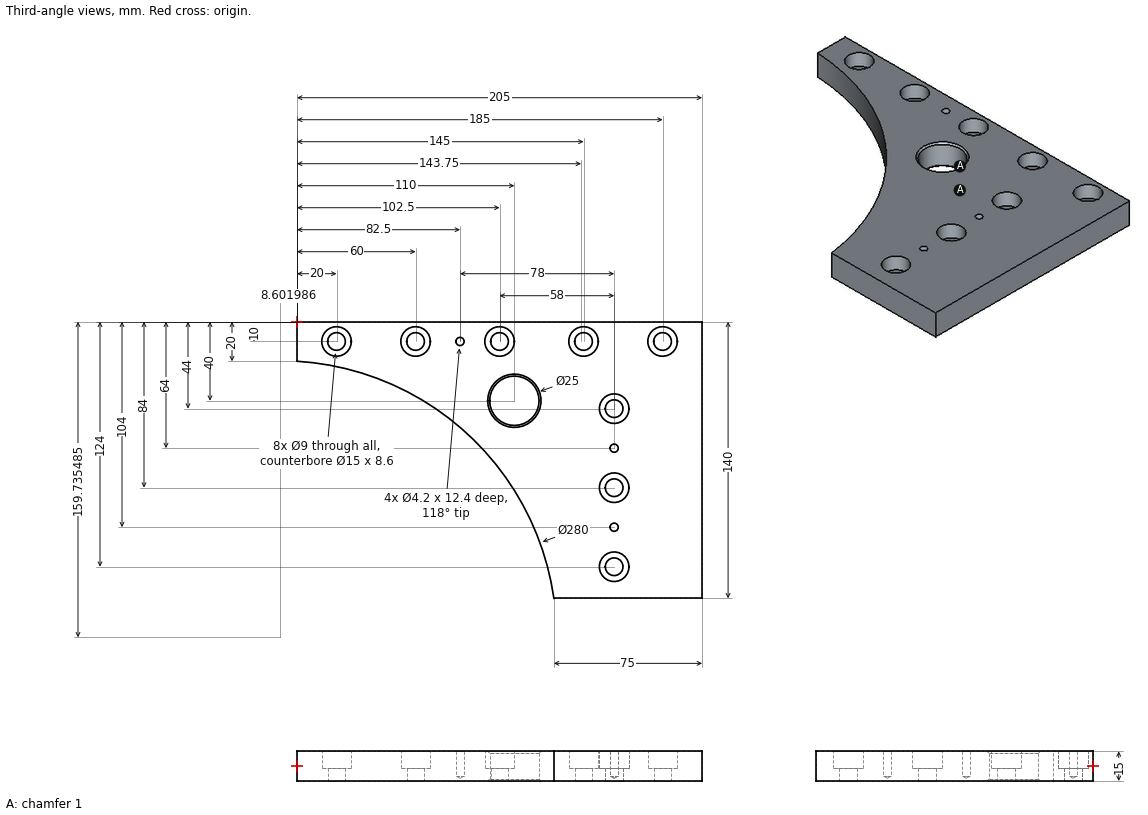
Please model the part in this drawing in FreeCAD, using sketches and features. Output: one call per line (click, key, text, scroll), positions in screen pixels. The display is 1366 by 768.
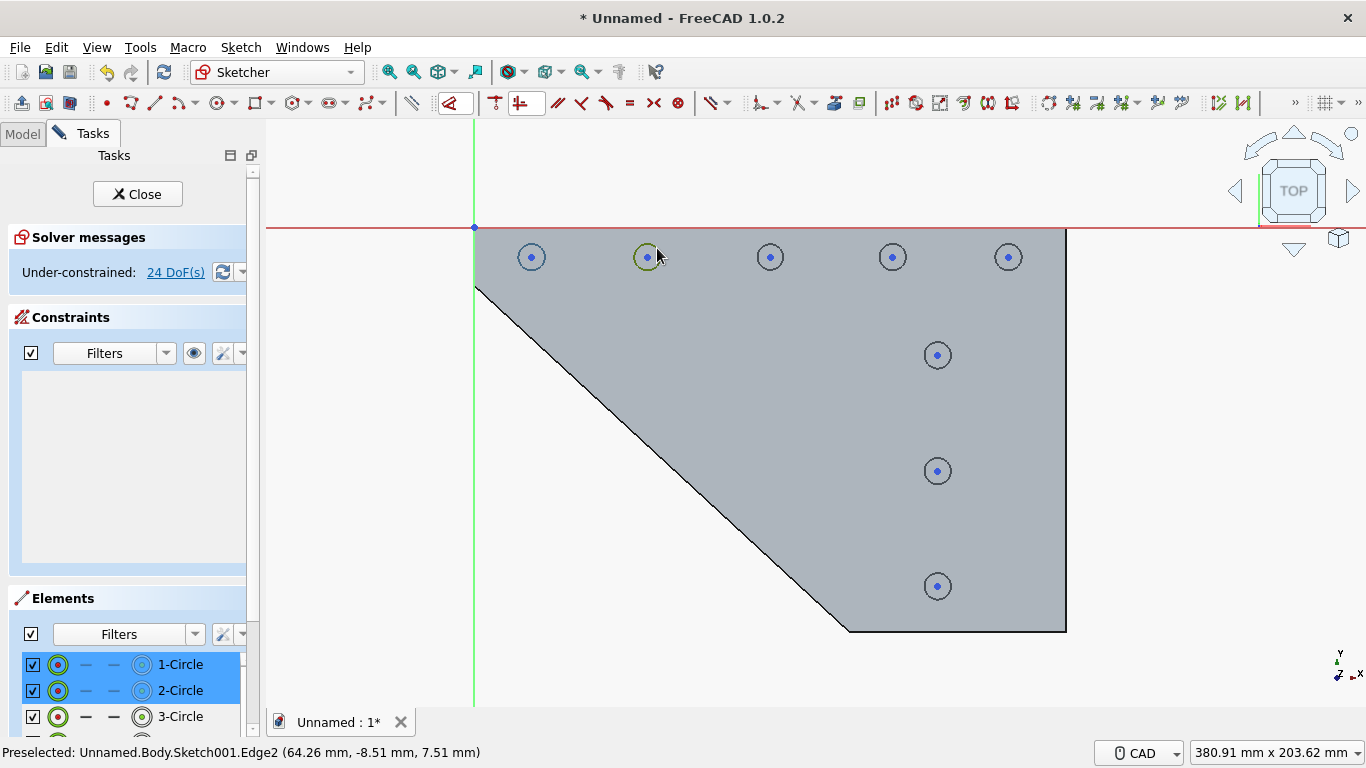
click(902, 248)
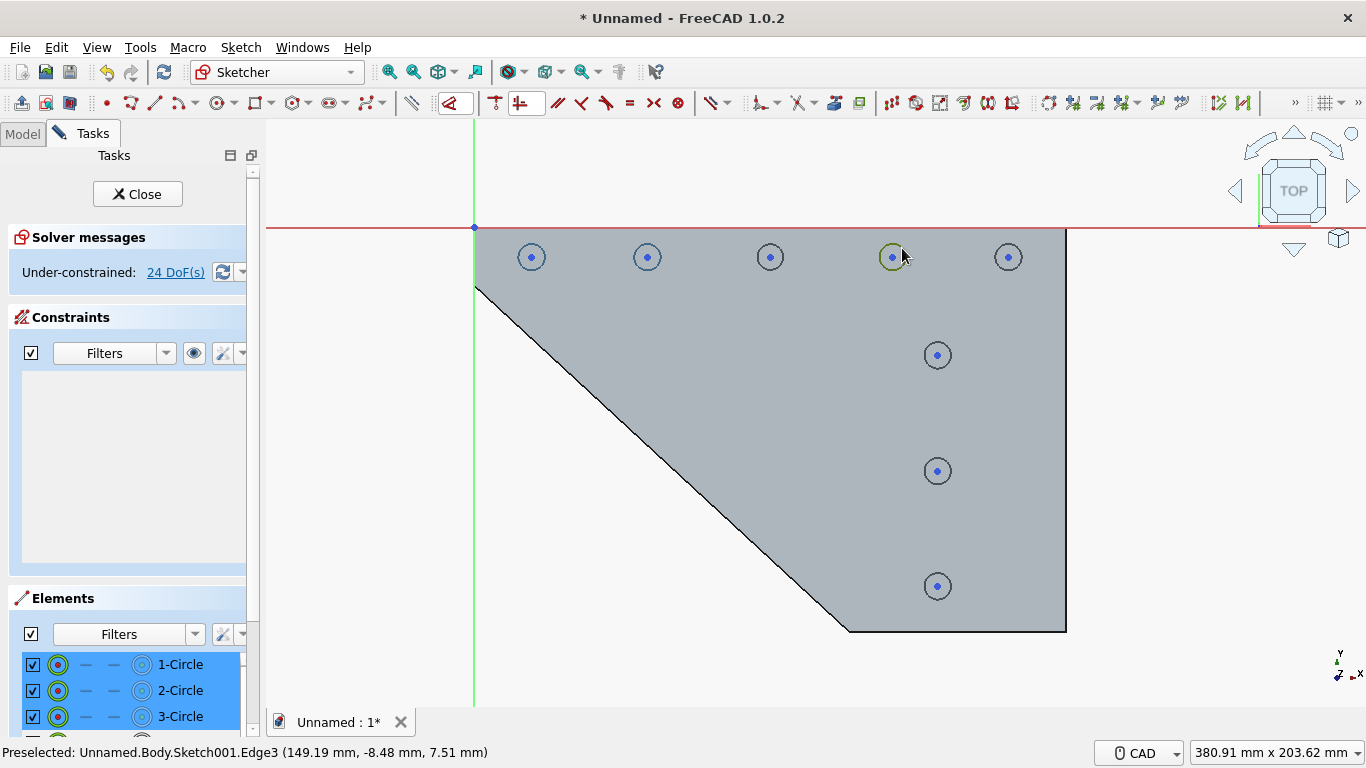
click(779, 248)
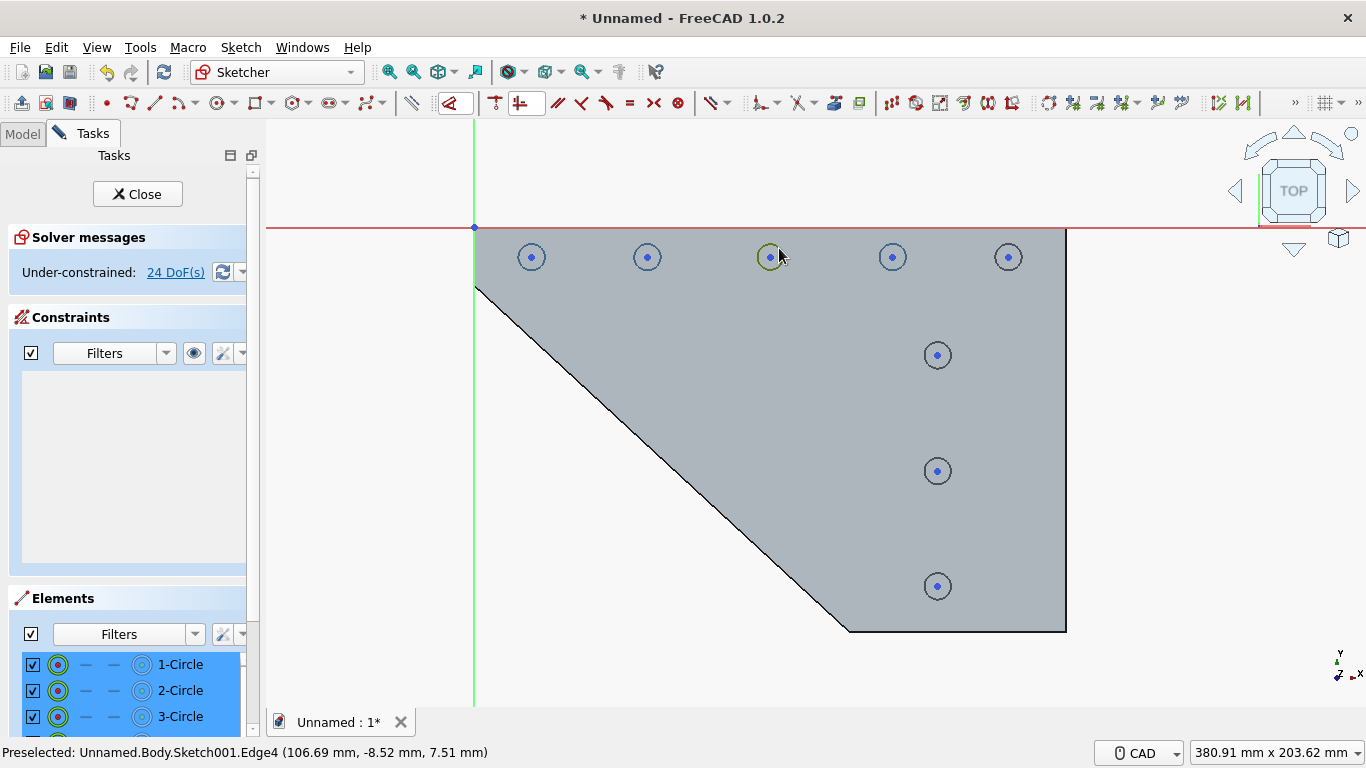
click(1018, 248)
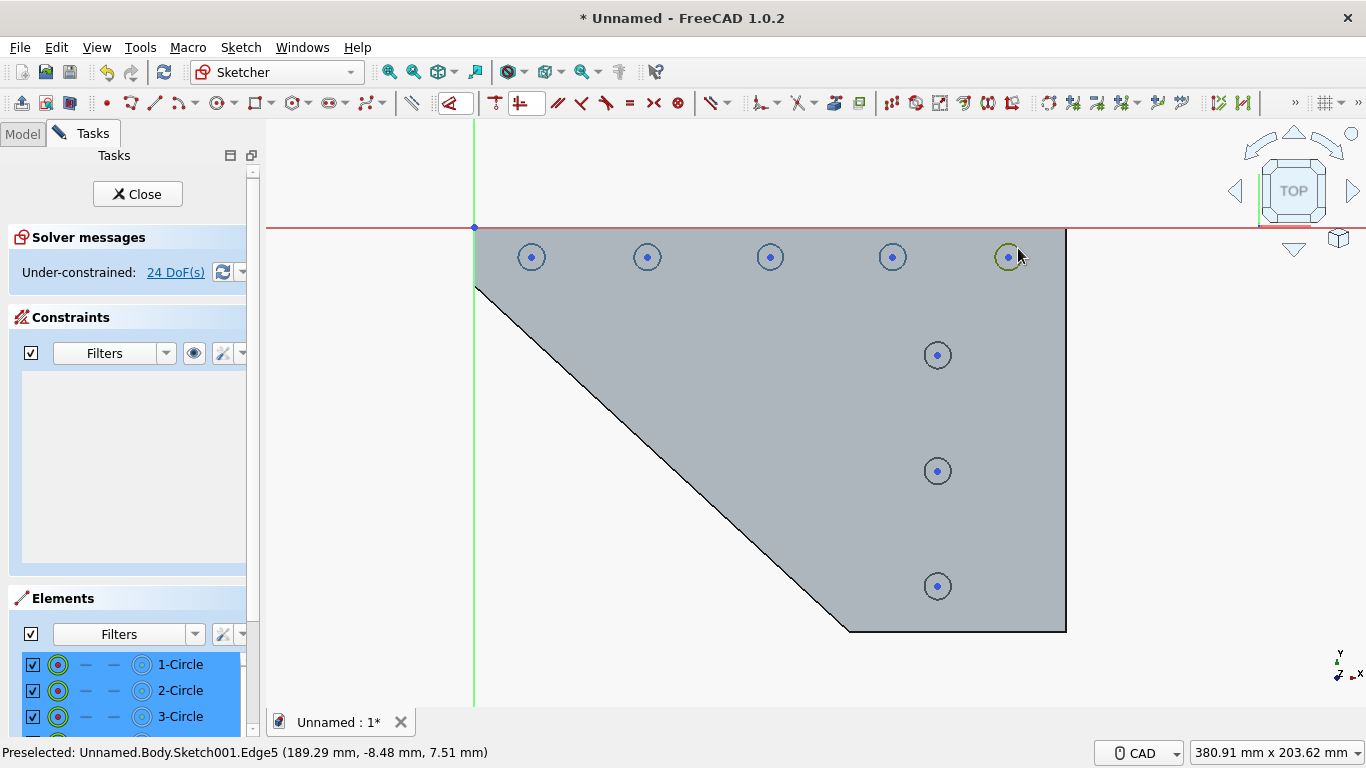
click(947, 346)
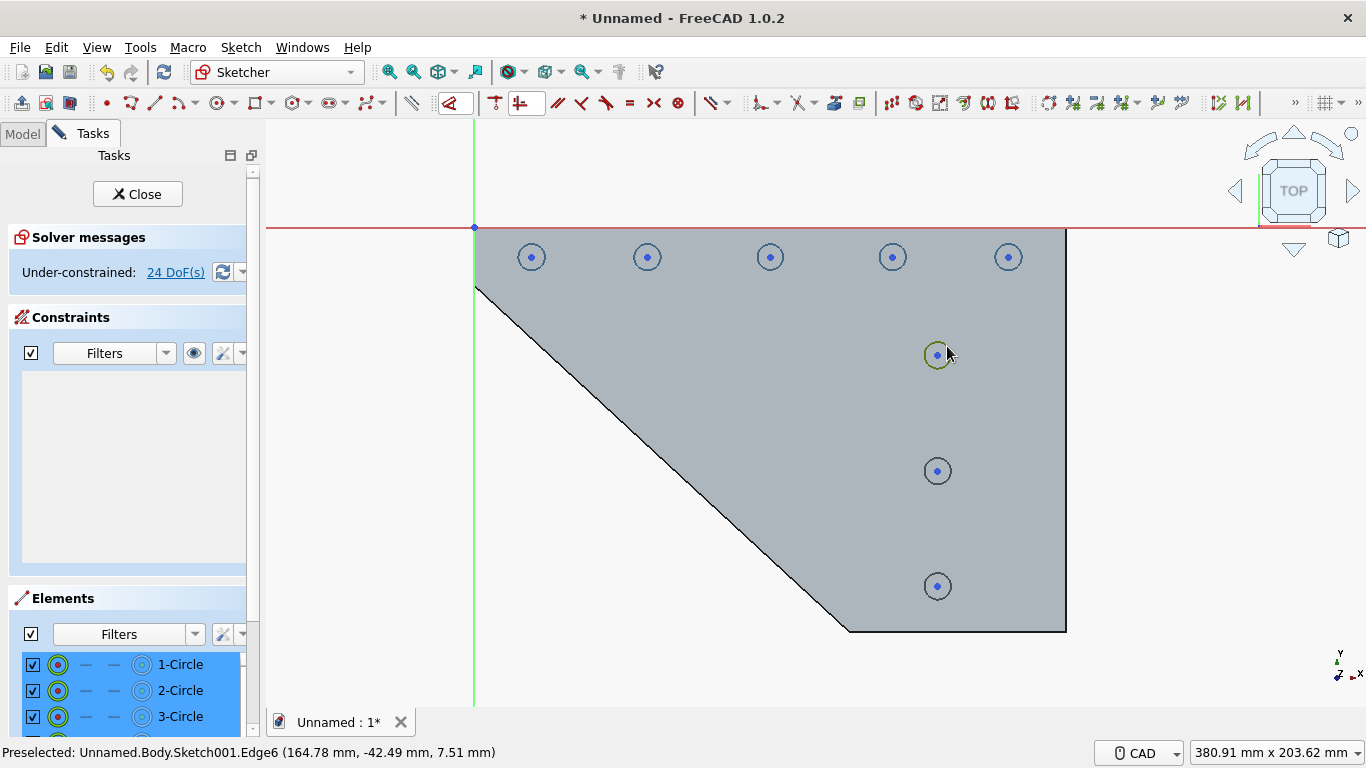
click(947, 462)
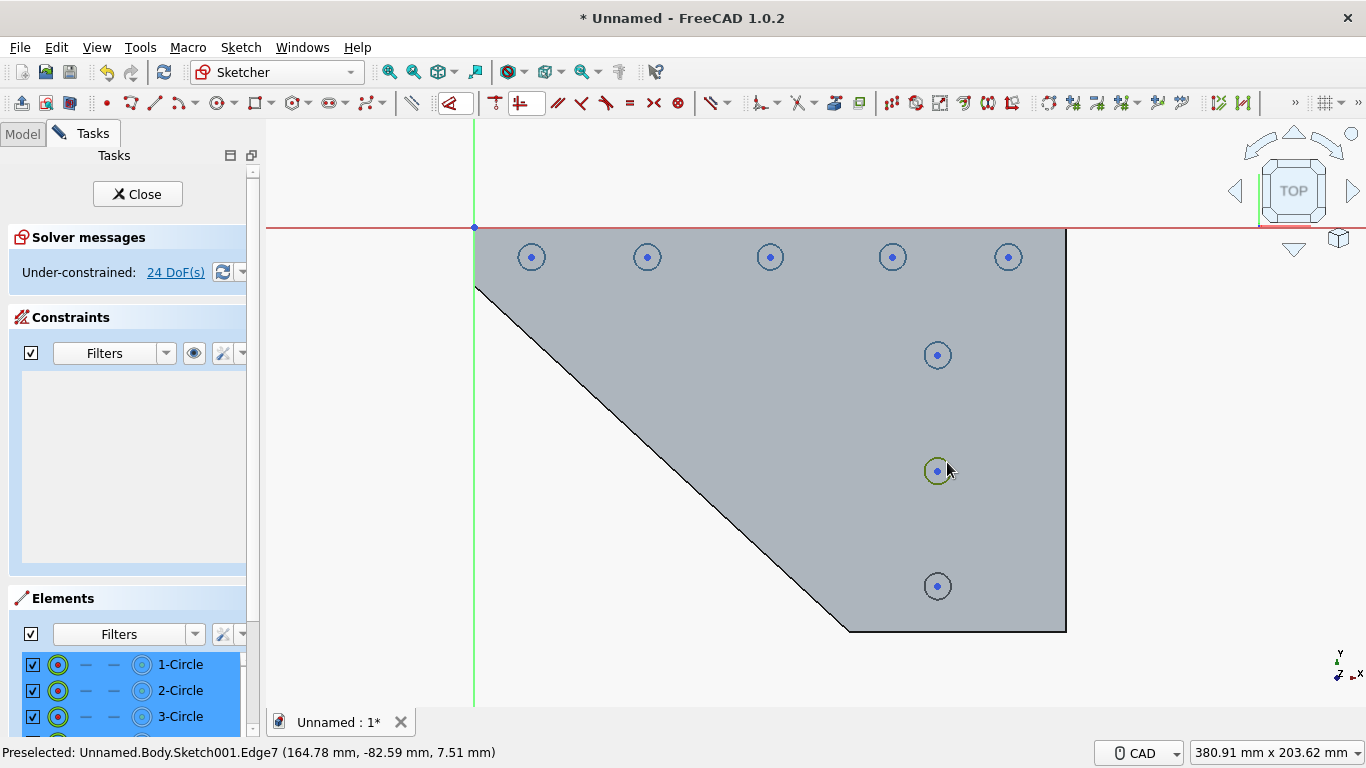
click(947, 577)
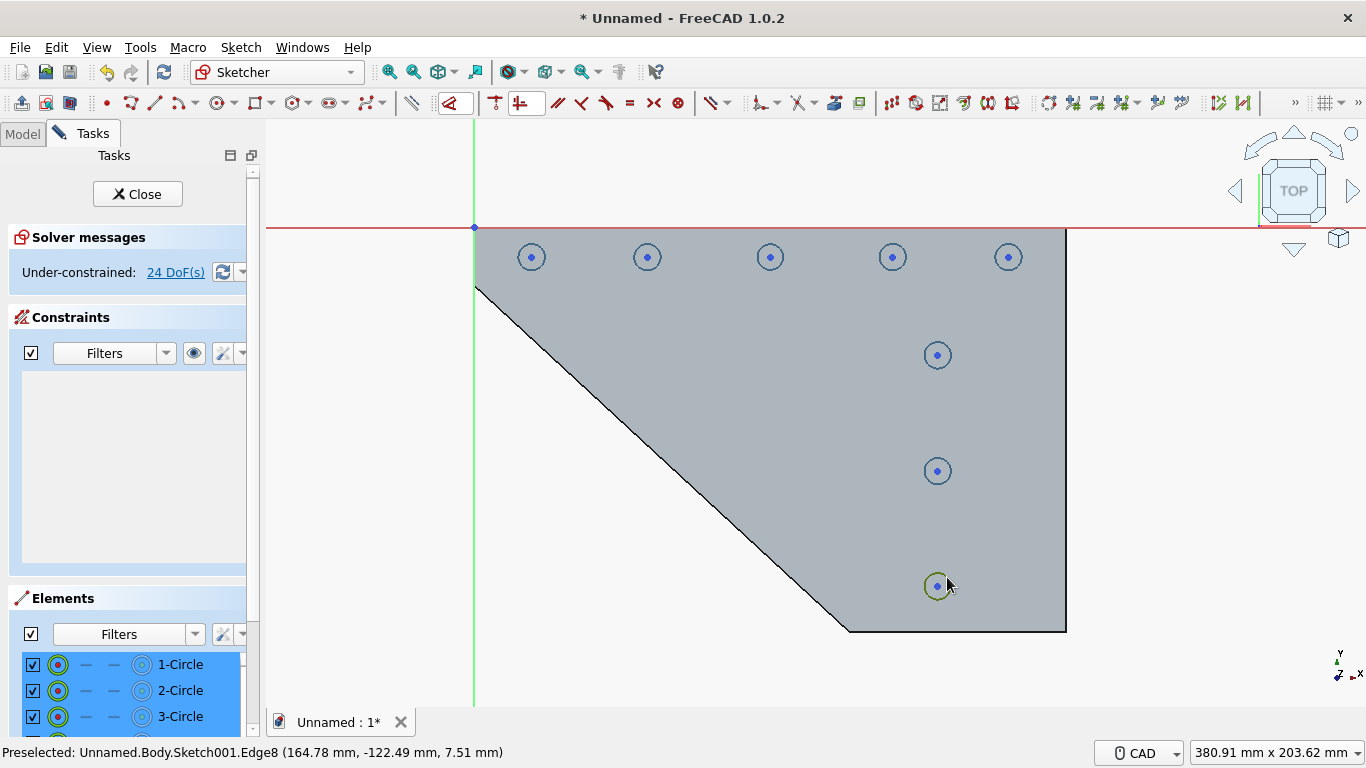
click(630, 104)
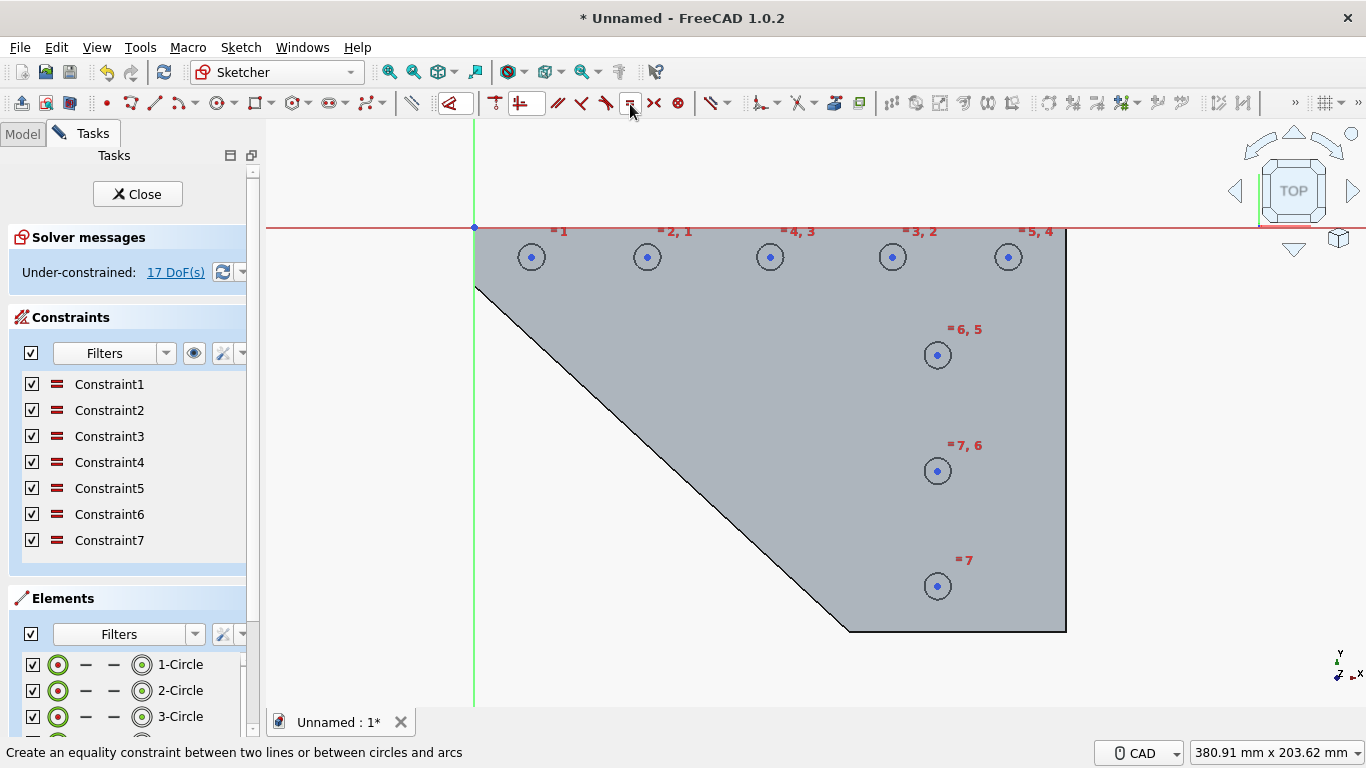
click(532, 257)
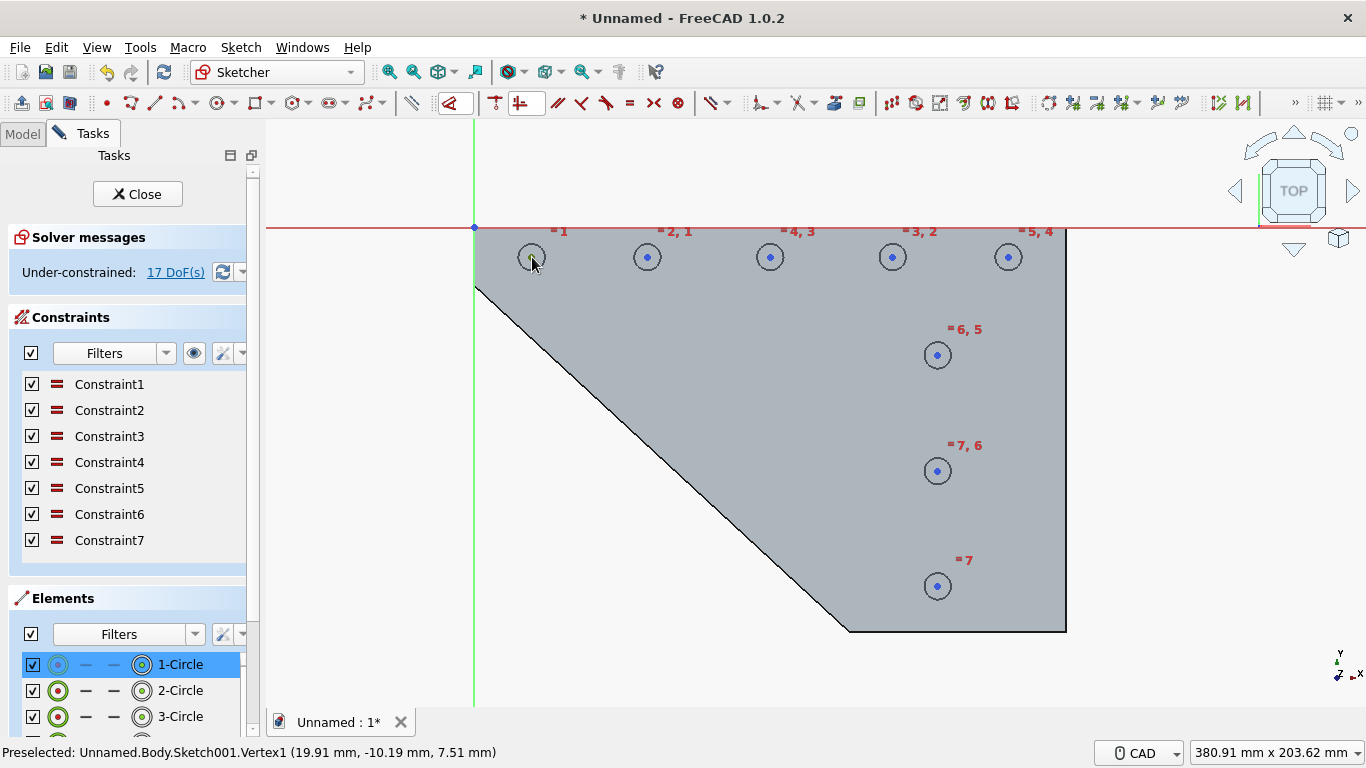
click(647, 257)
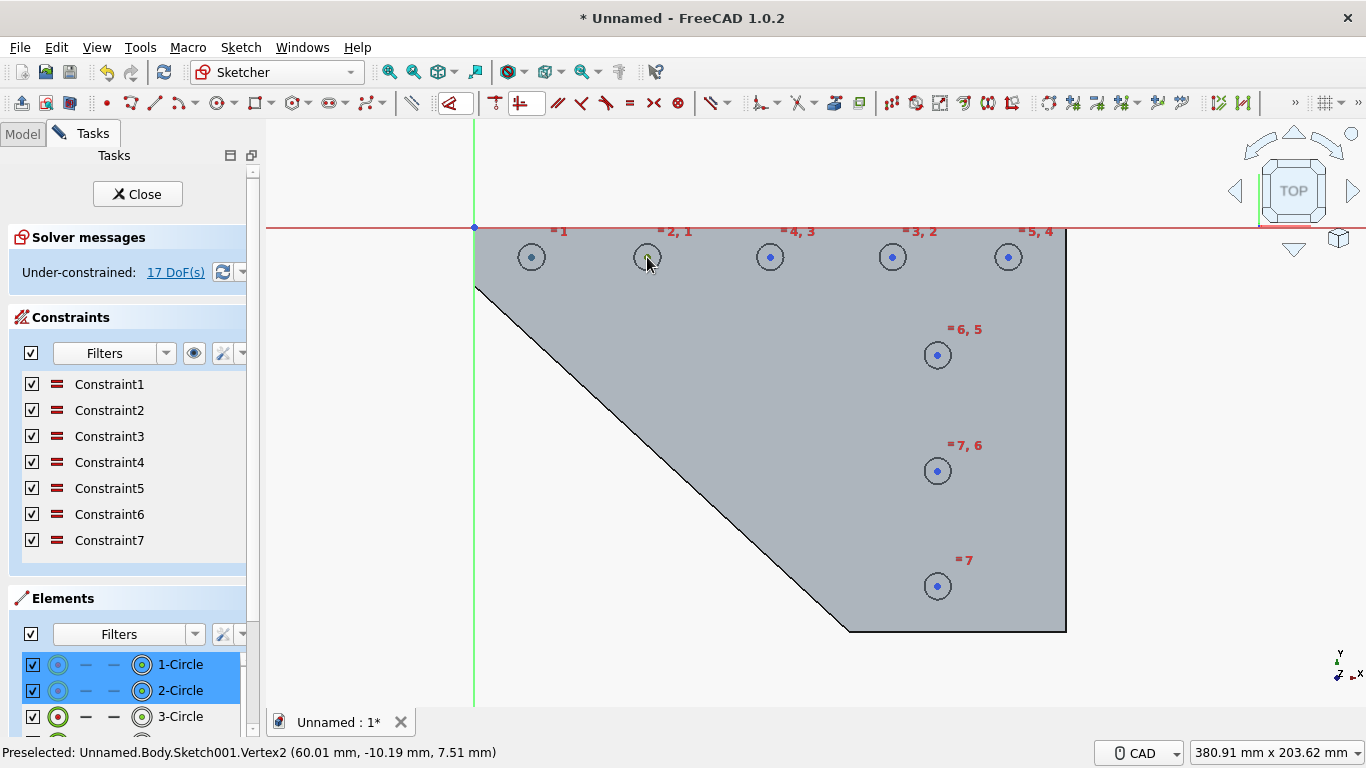
click(540, 104)